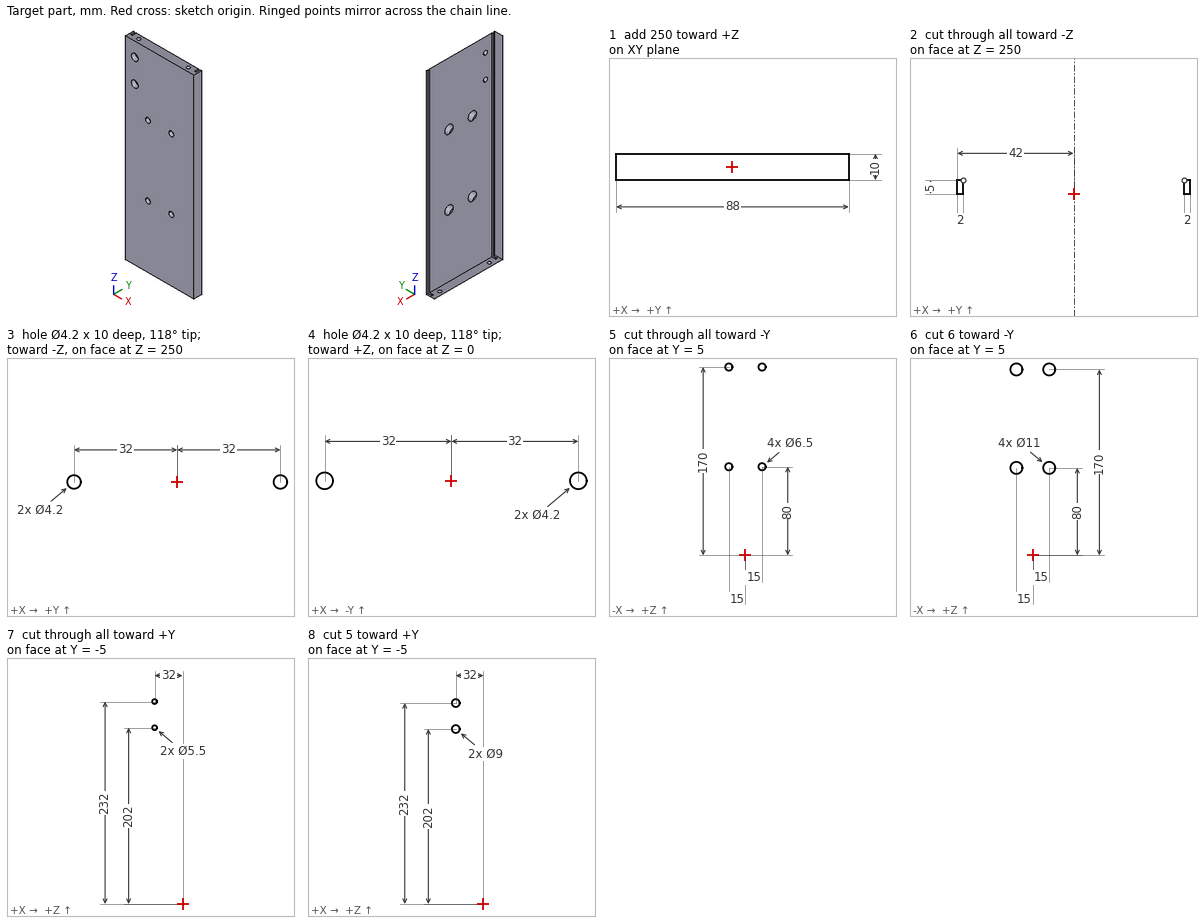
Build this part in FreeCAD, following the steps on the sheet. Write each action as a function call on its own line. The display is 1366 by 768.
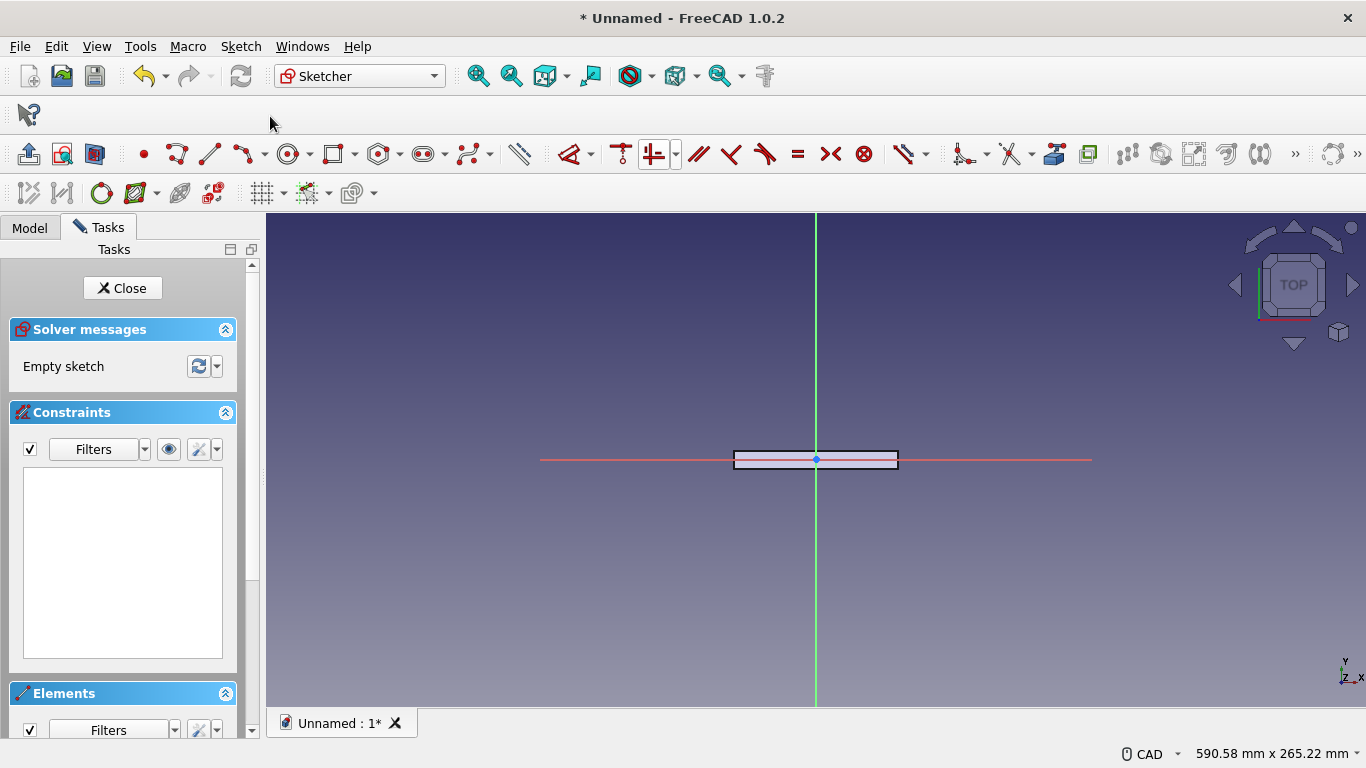
scroll(838, 454, up, 7)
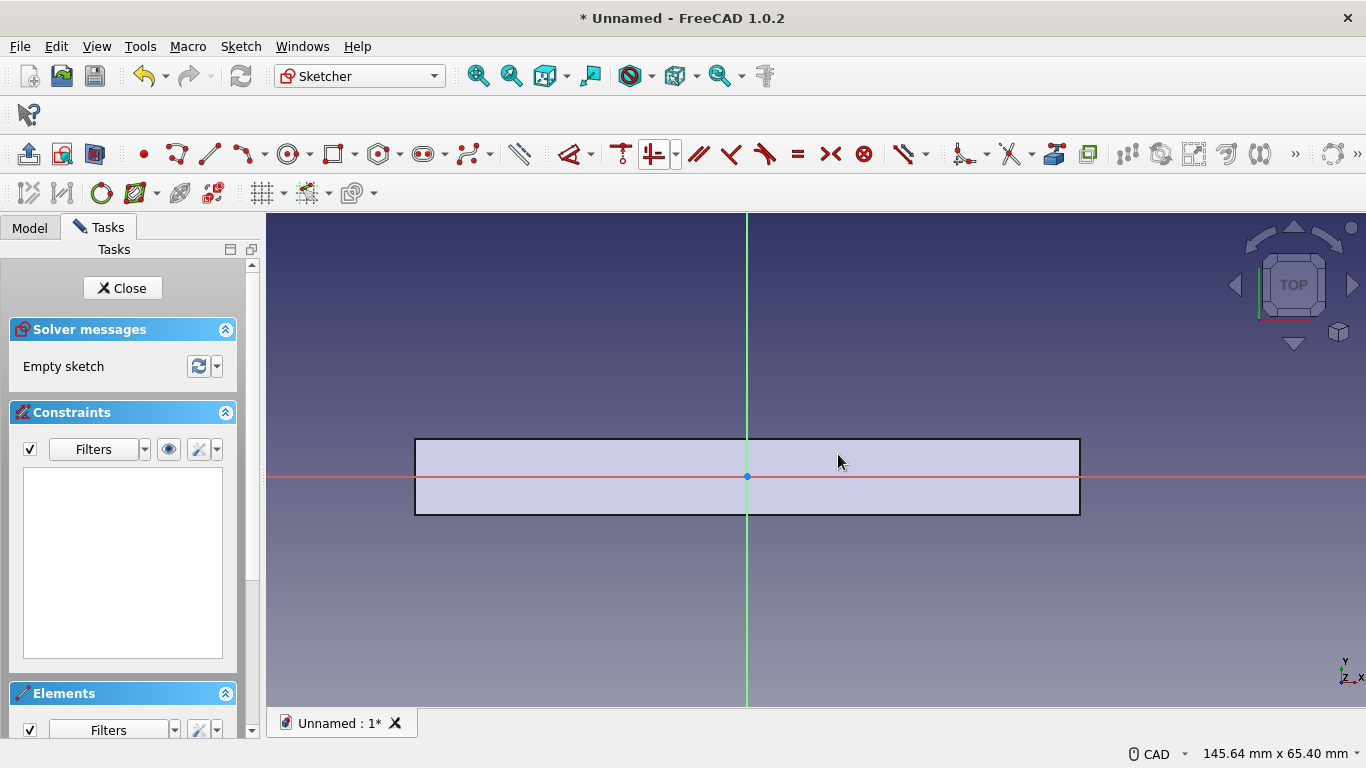
click(332, 154)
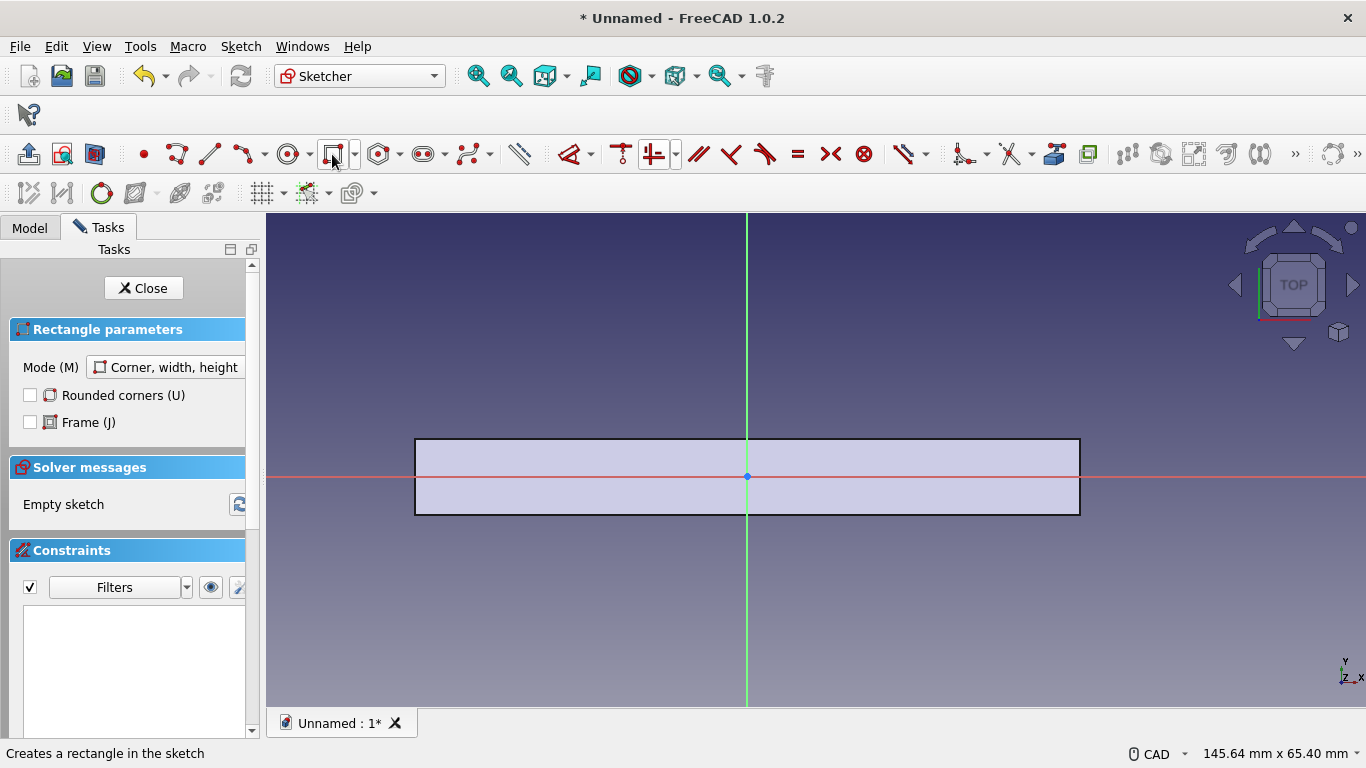
click(430, 439)
click(445, 477)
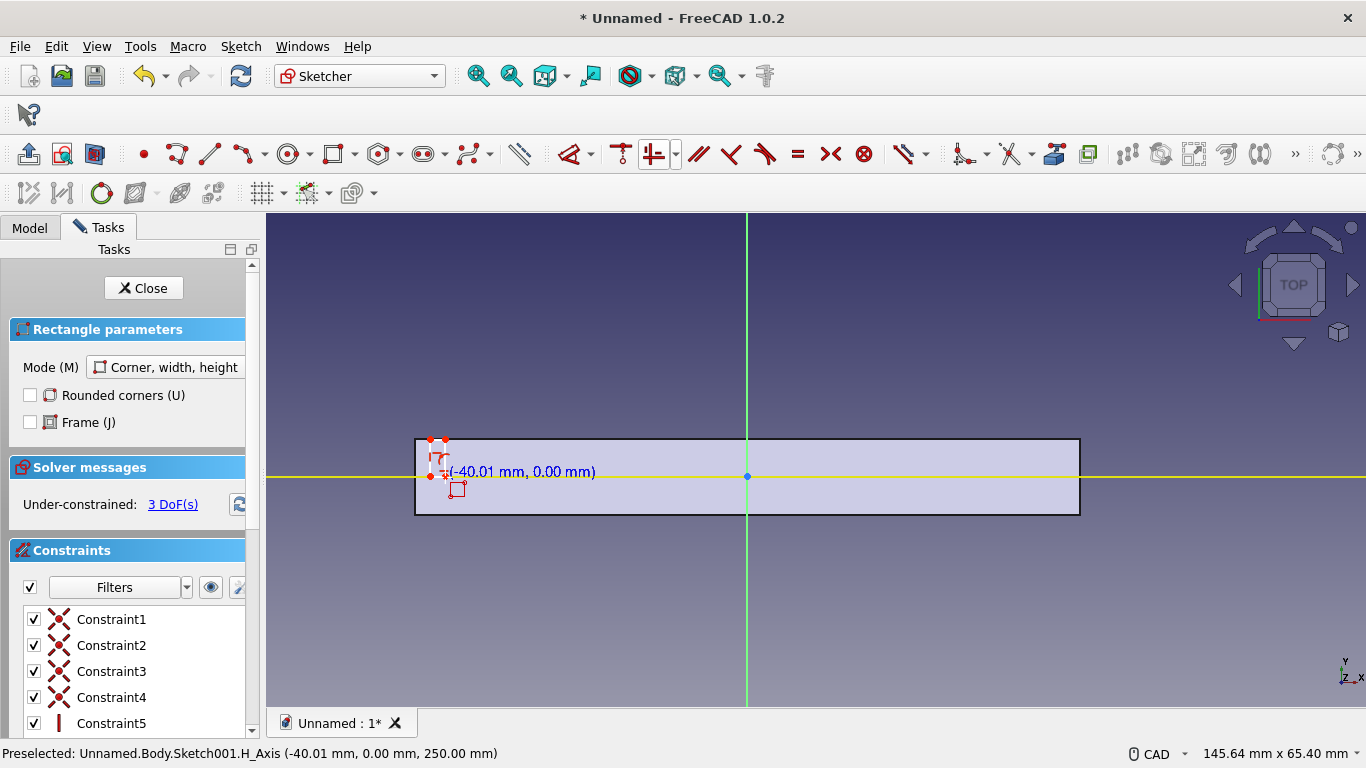
click(1049, 439)
click(1064, 477)
key(Escape)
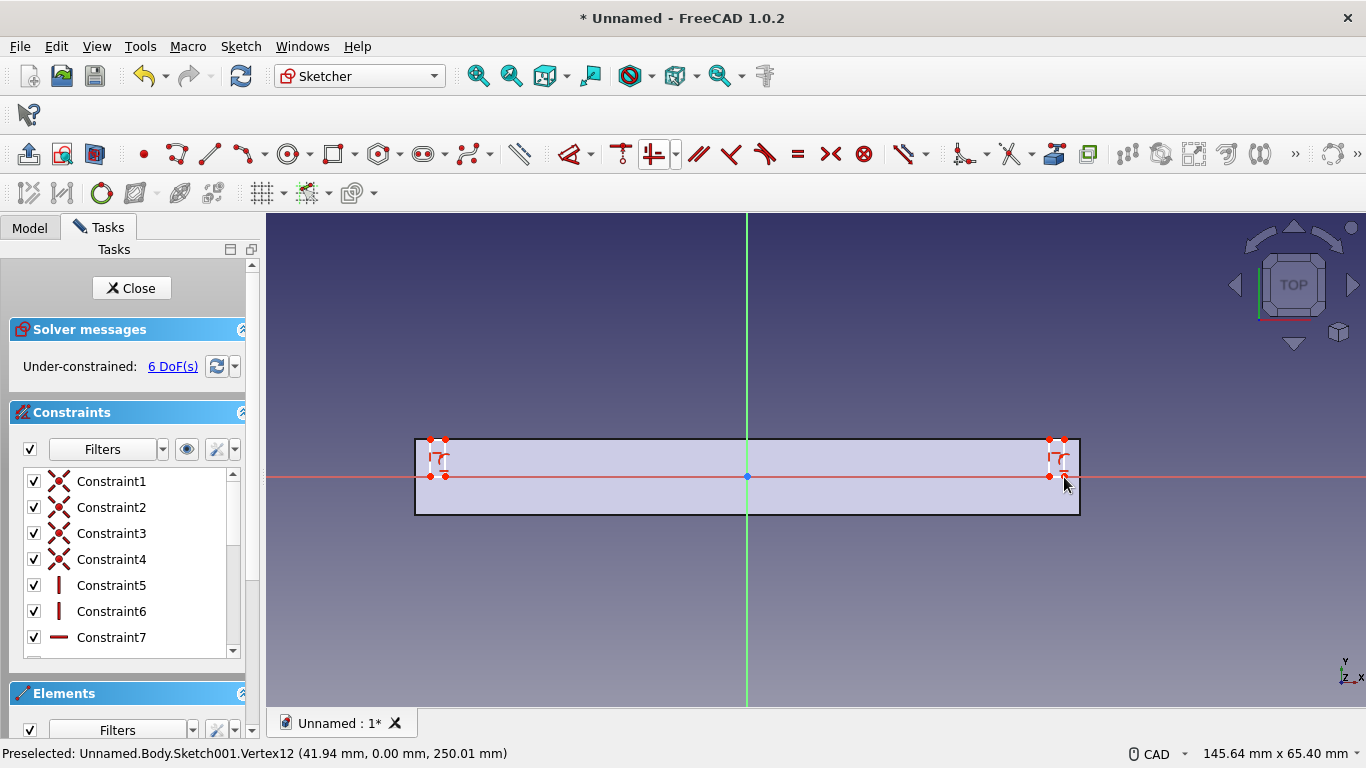
click(445, 440)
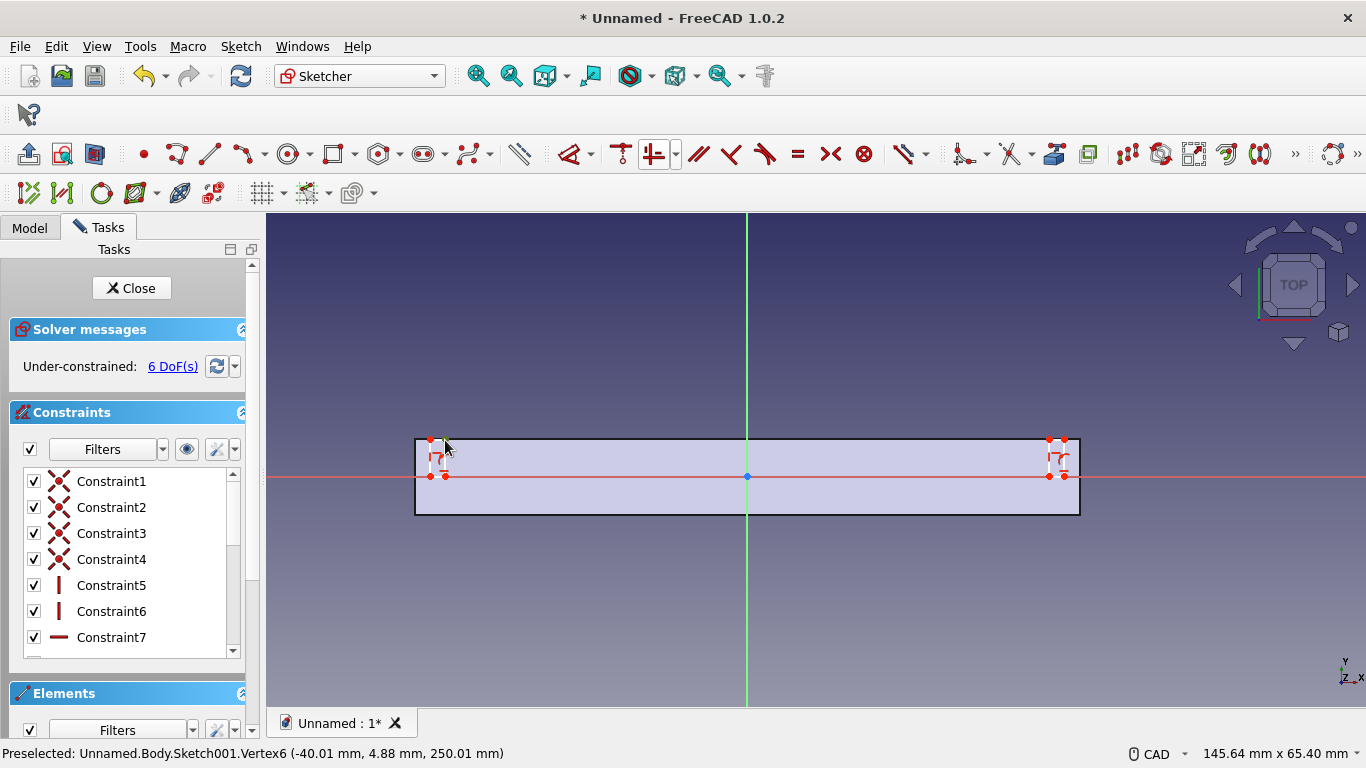
click(1049, 440)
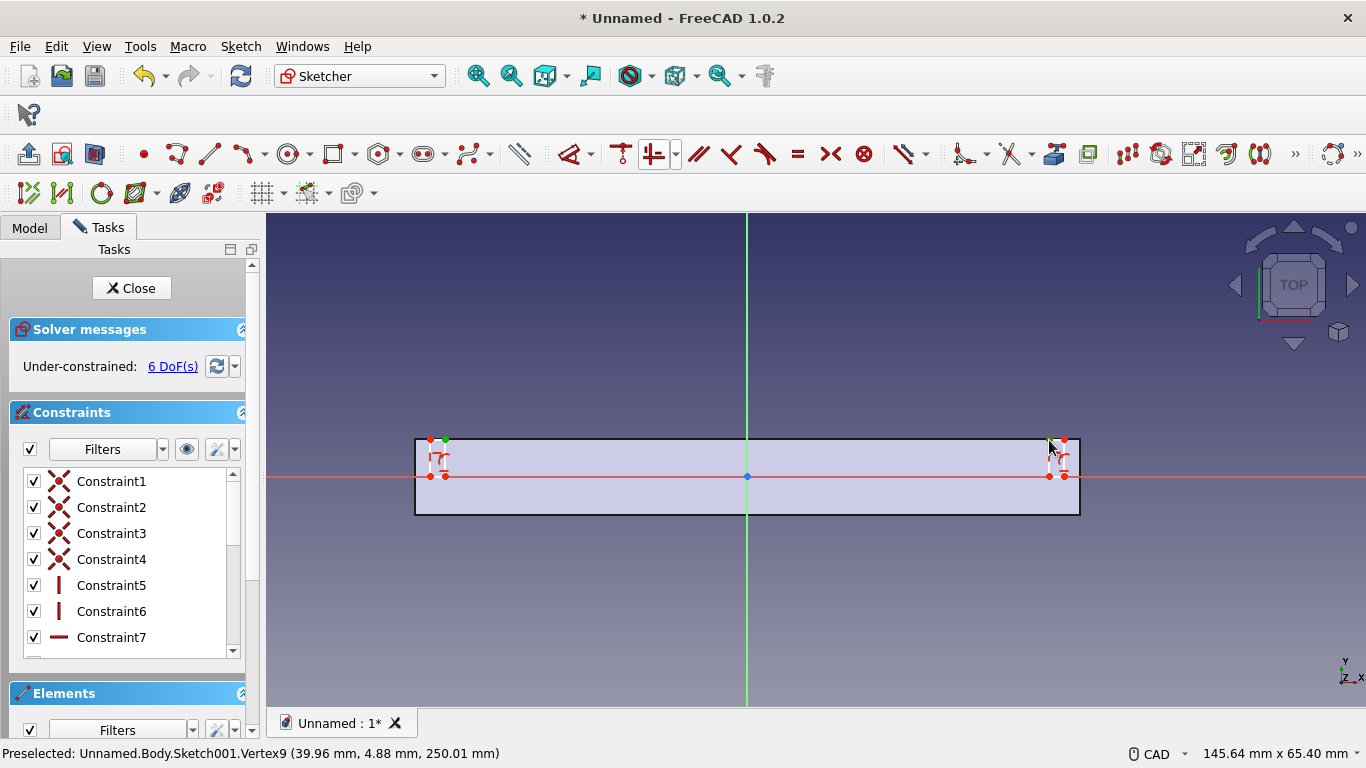
click(747, 648)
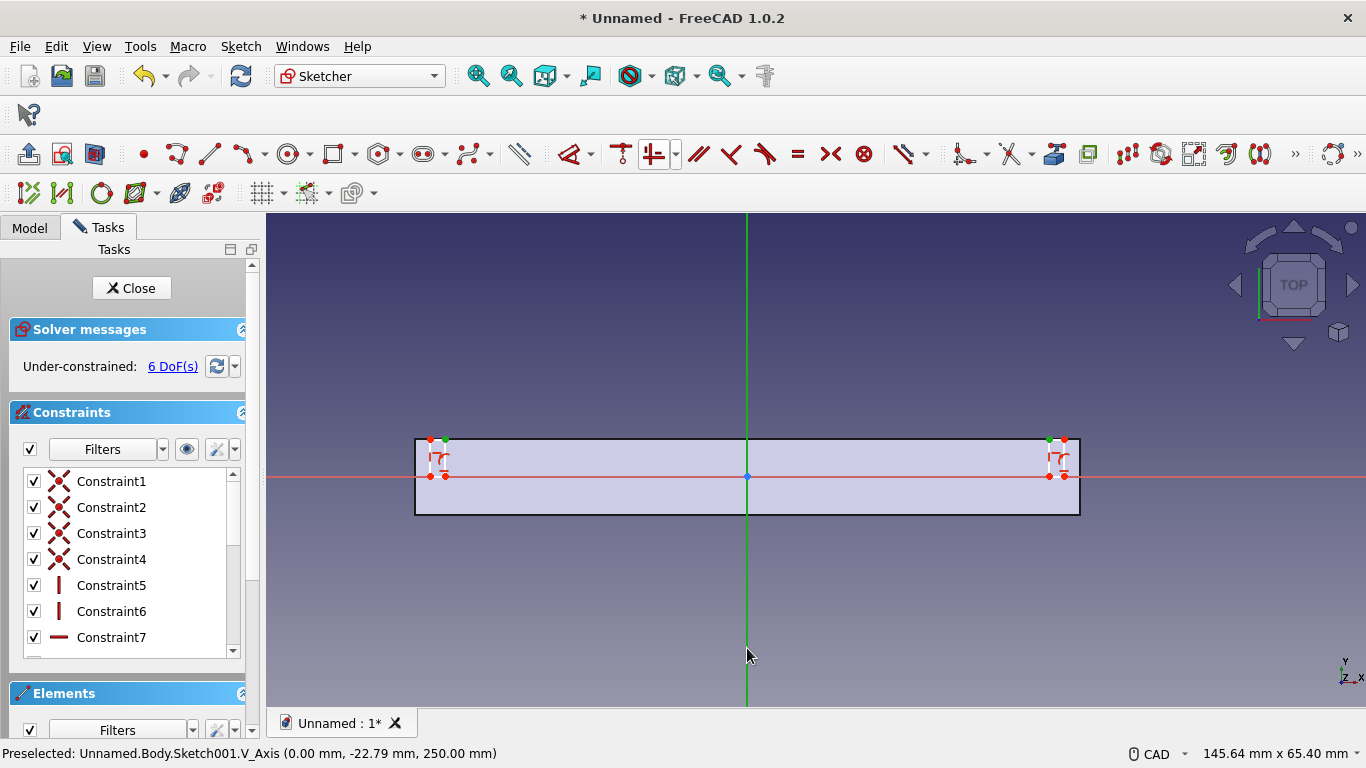
click(831, 154)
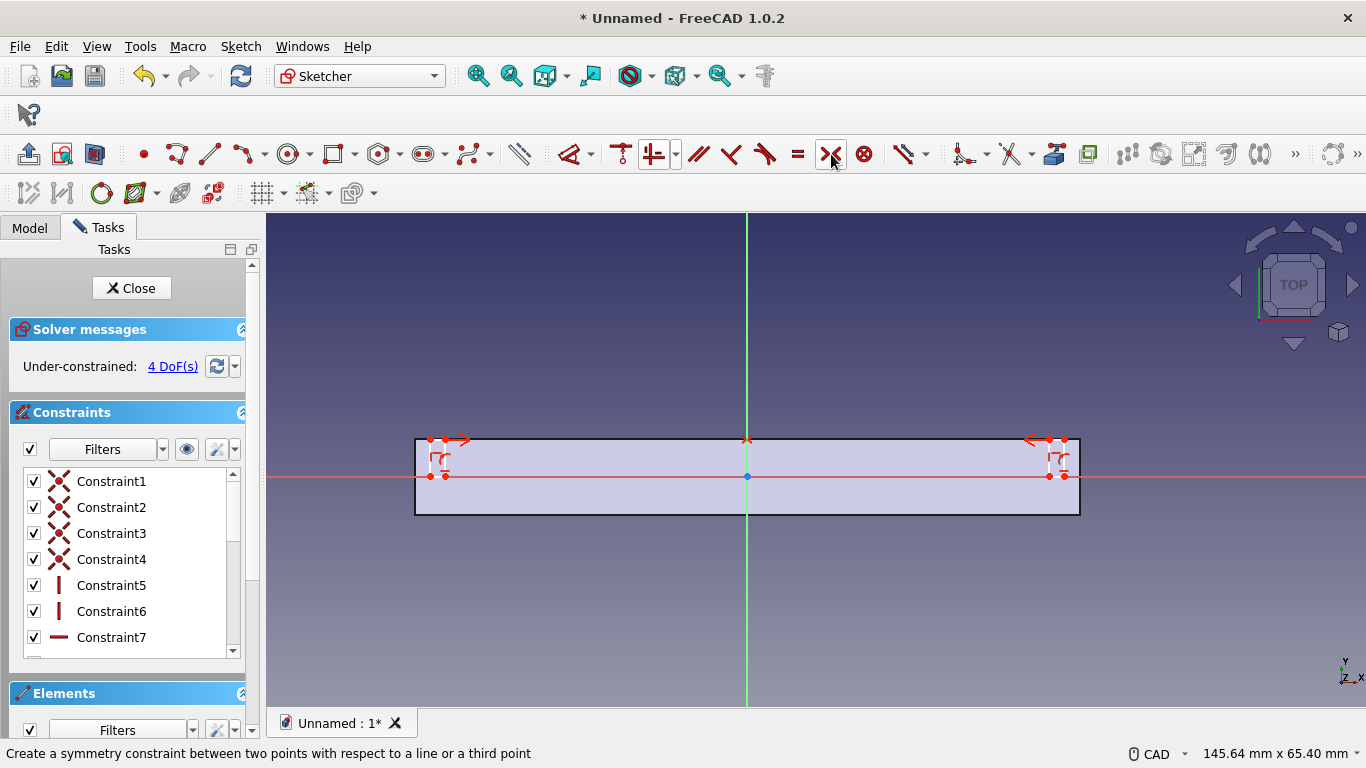
click(568, 154)